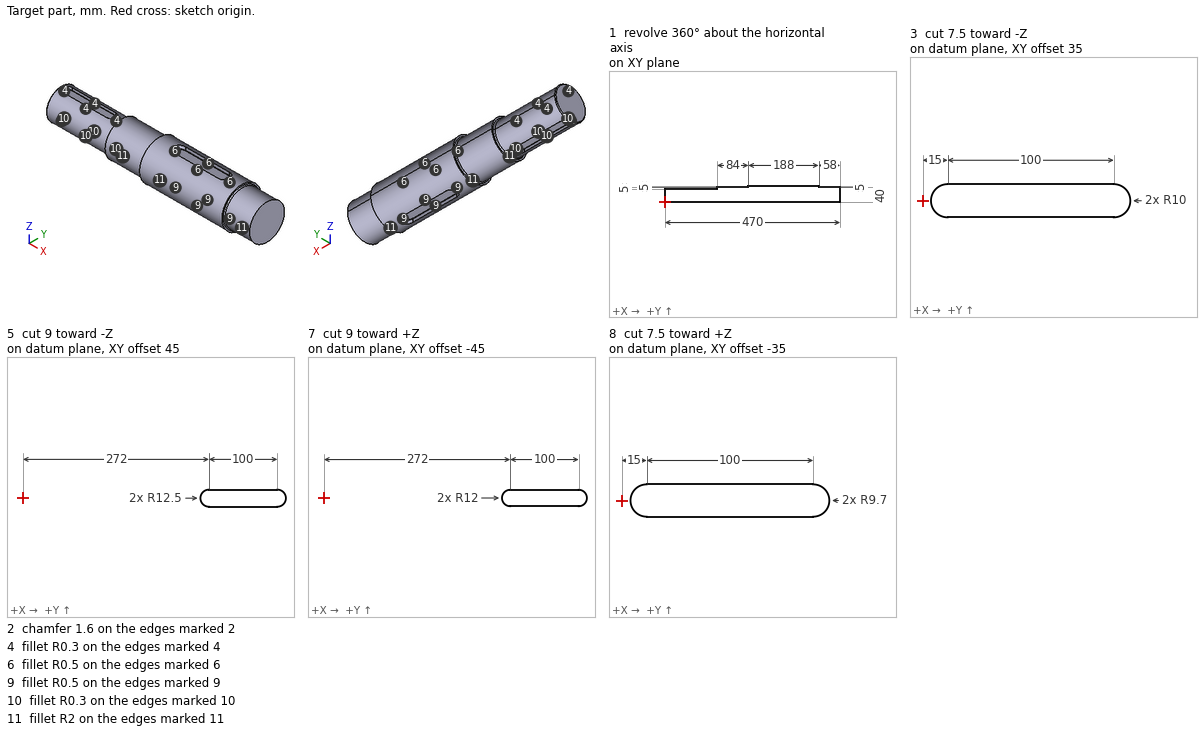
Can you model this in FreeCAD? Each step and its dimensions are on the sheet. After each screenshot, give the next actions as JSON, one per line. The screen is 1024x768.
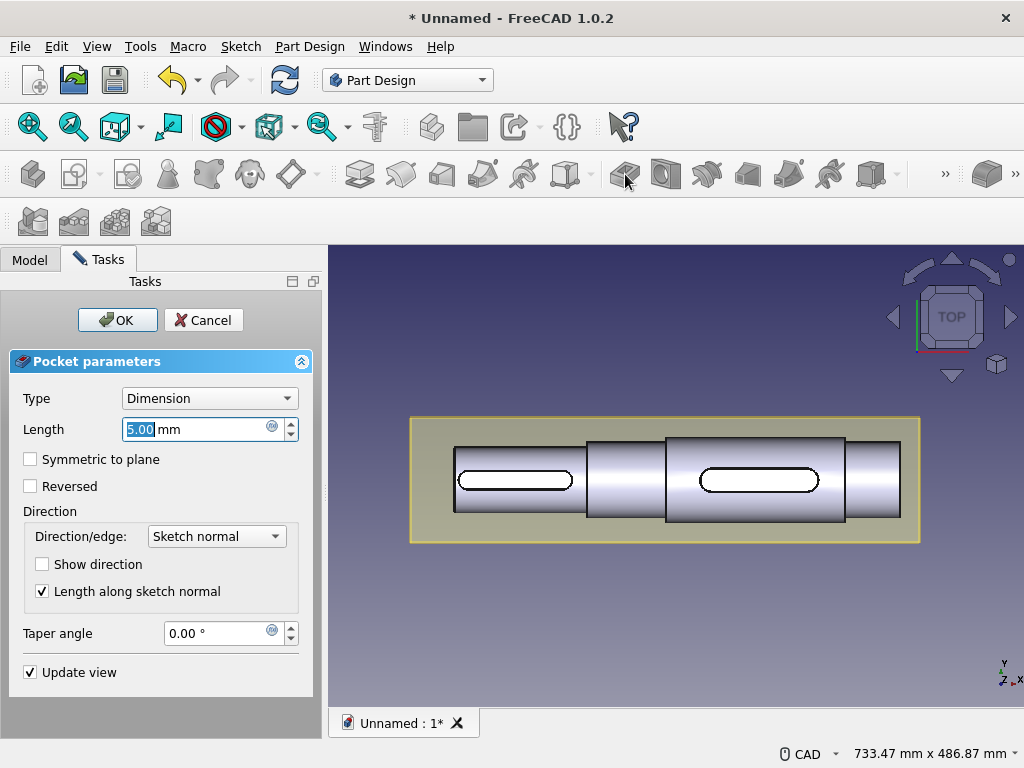
{"action": "type", "text": "9"}
{"action": "key", "text": "Tab"}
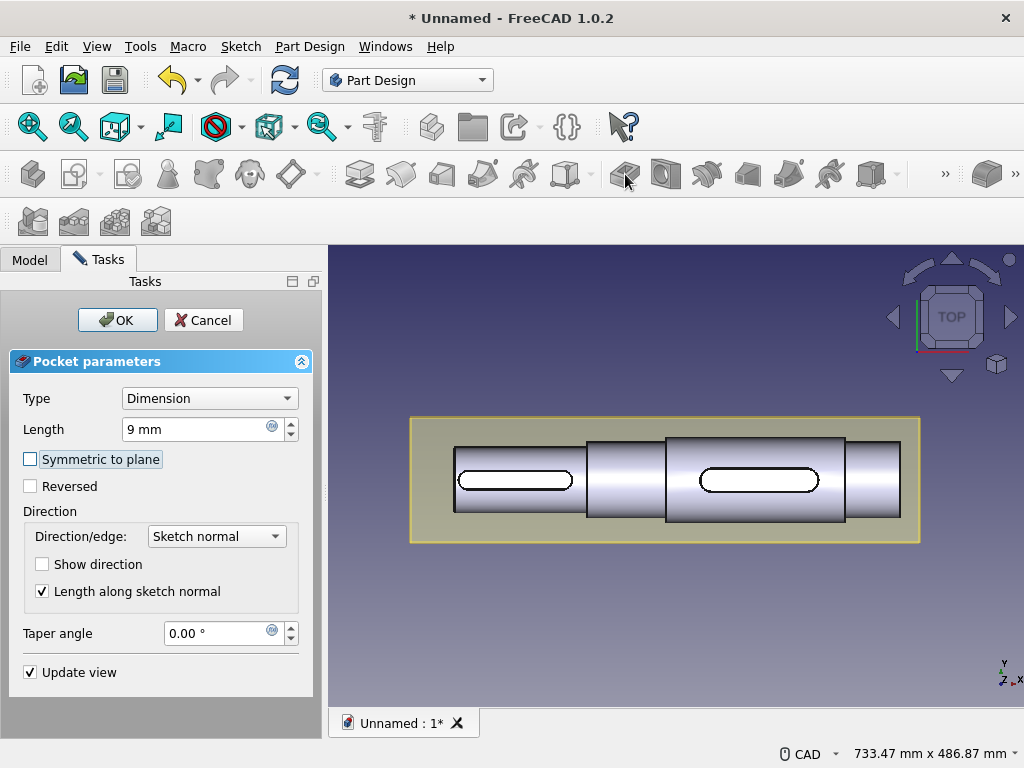
{"action": "left_click", "coordinate": [31, 486]}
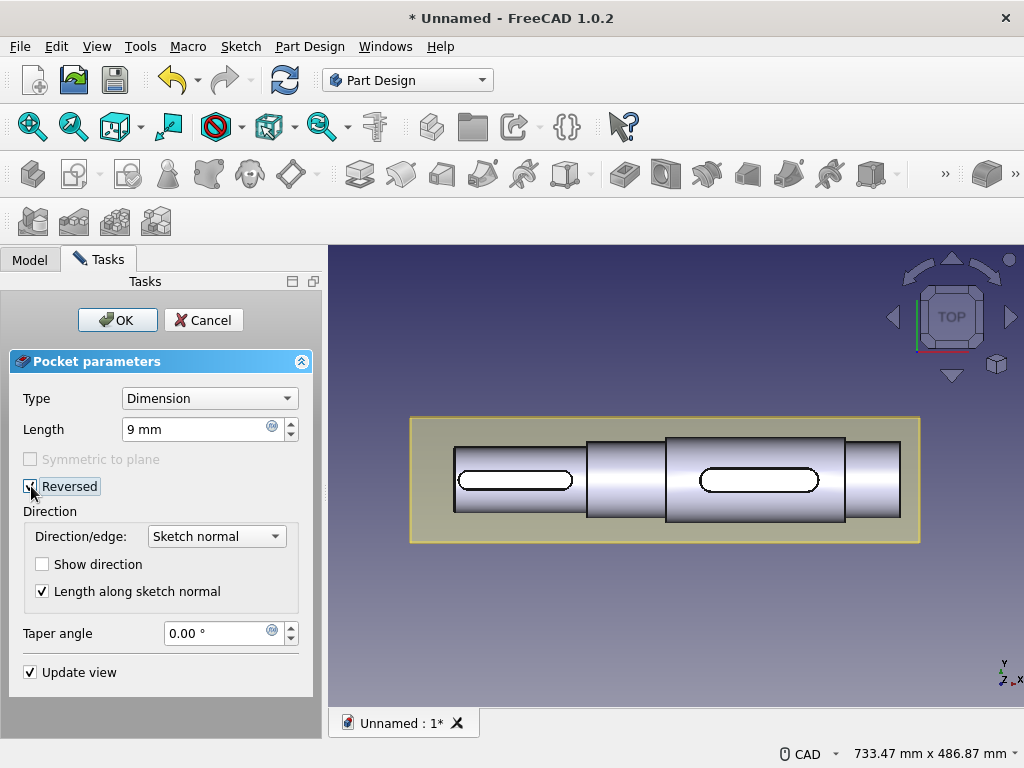
{"action": "left_click", "coordinate": [118, 320]}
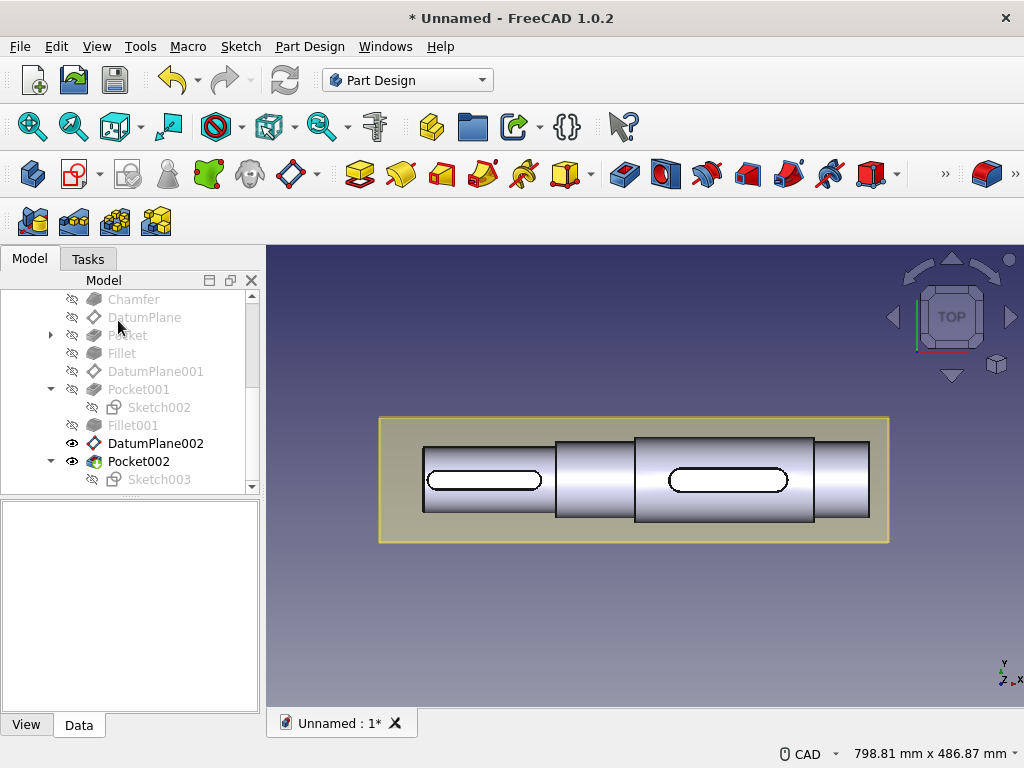
{"action": "left_click", "coordinate": [117, 443]}
{"action": "key", "text": "space"}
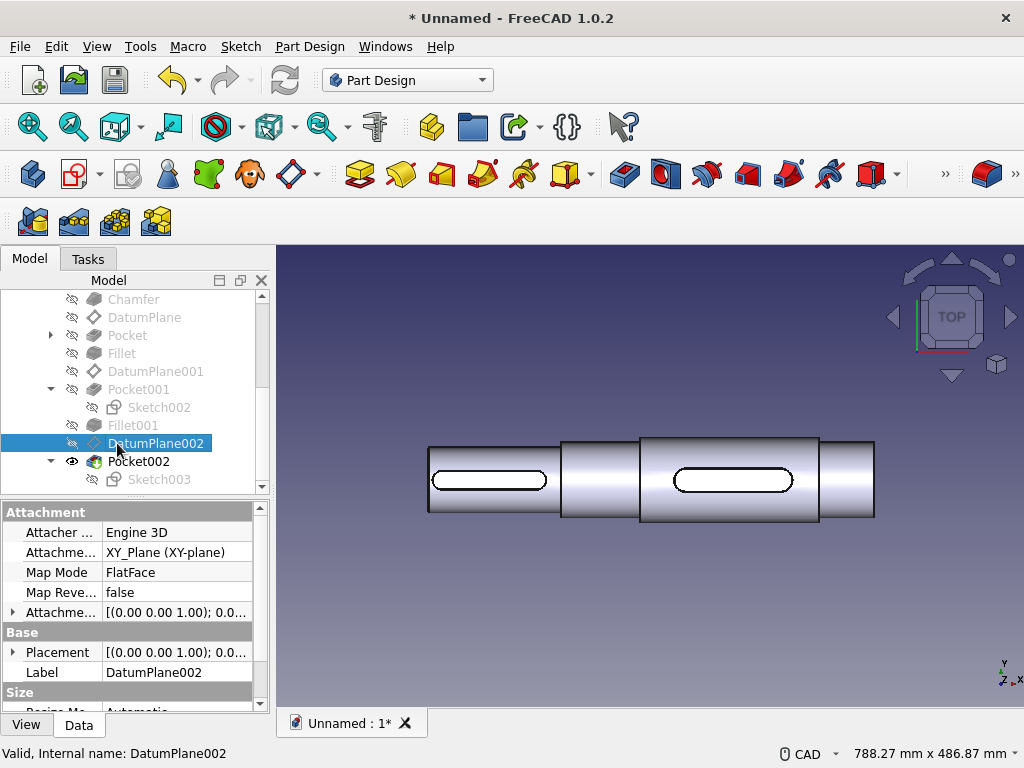
{"action": "scroll", "coordinate": [141, 385], "scroll_direction": "down", "scroll_amount": 3}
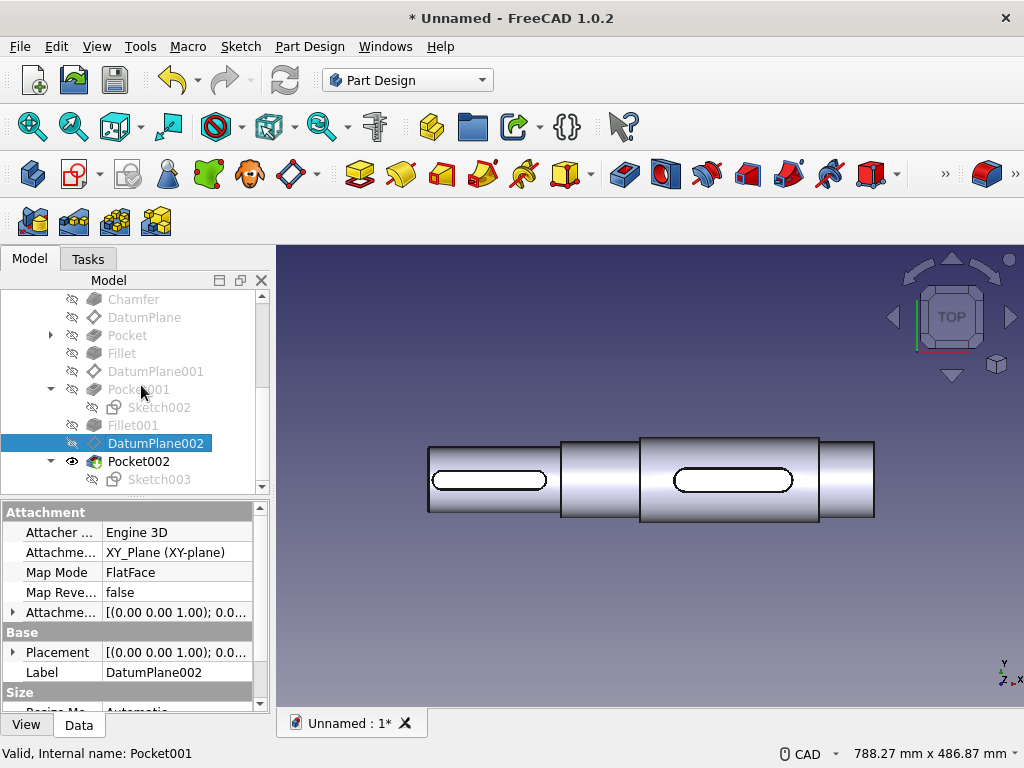
{"action": "scroll", "coordinate": [141, 385], "scroll_direction": "up", "scroll_amount": 15}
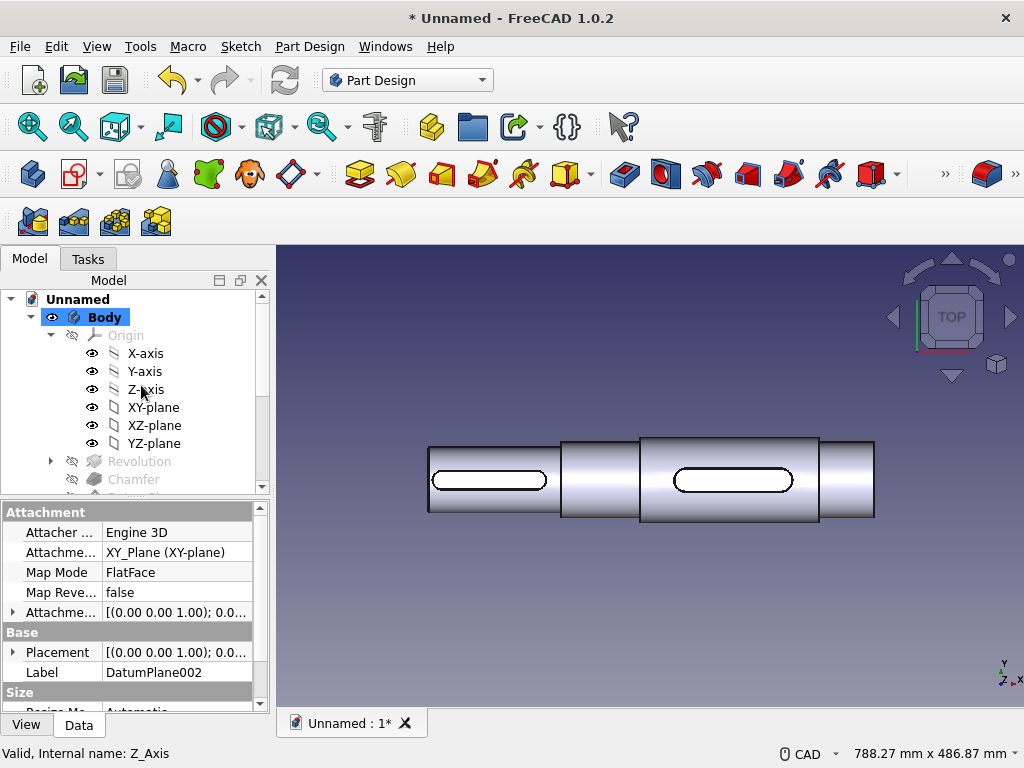
{"action": "left_click", "coordinate": [137, 407]}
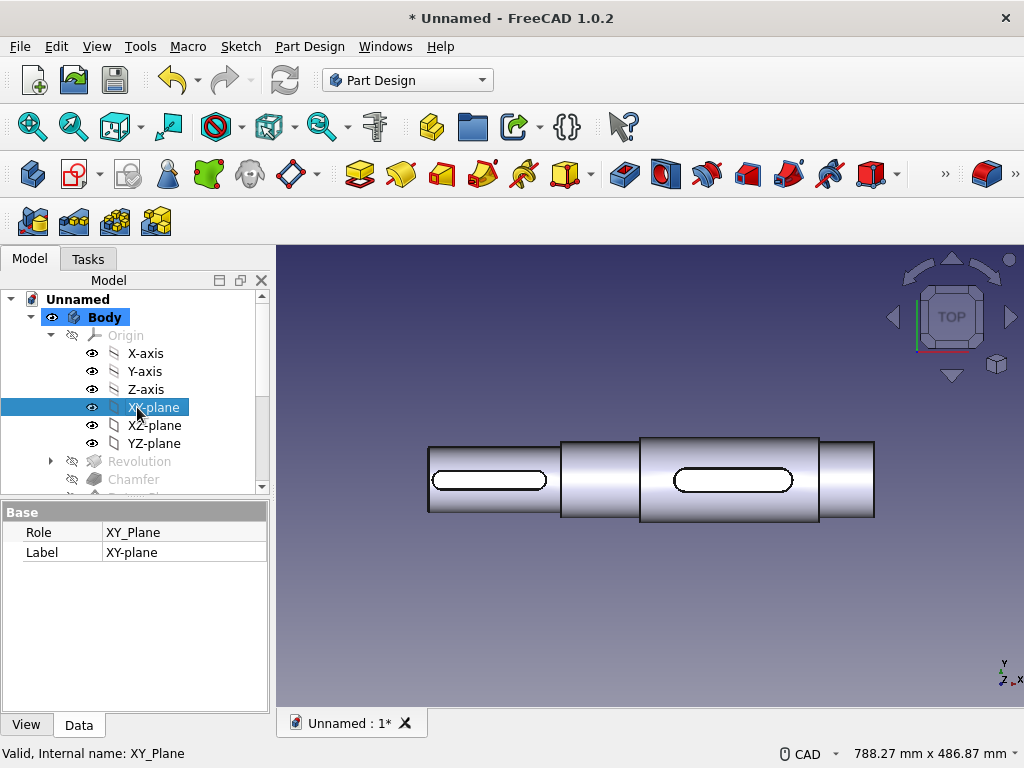
{"action": "left_click", "coordinate": [290, 174]}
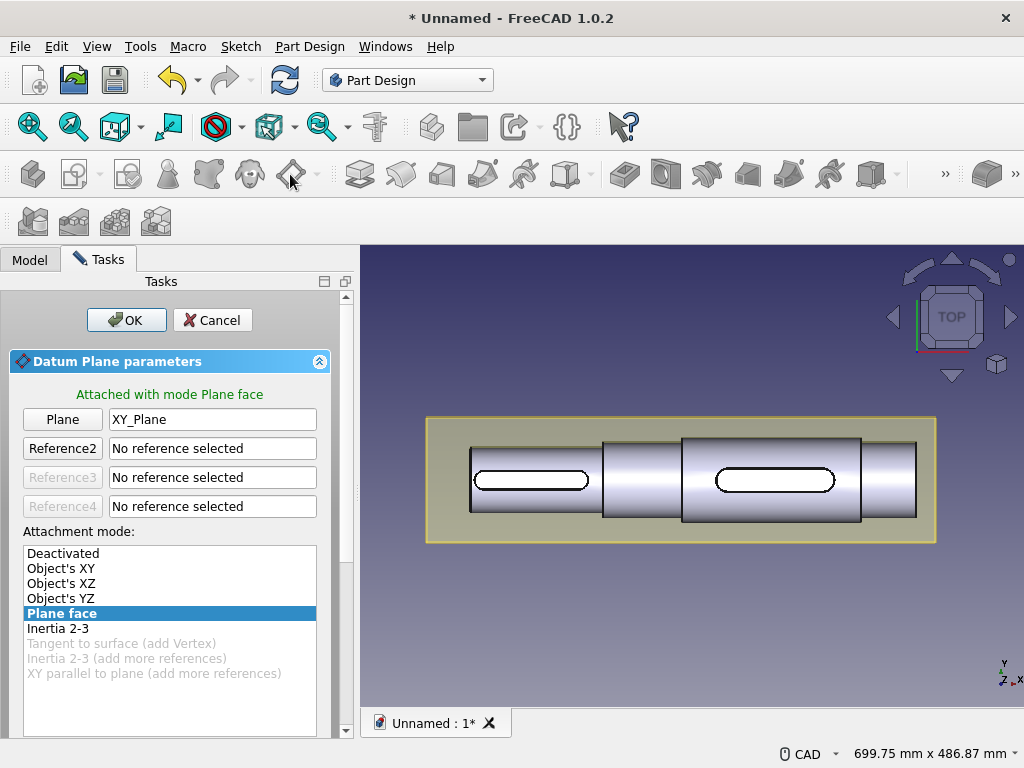
{"action": "scroll", "coordinate": [346, 514], "scroll_direction": "down", "scroll_amount": 4}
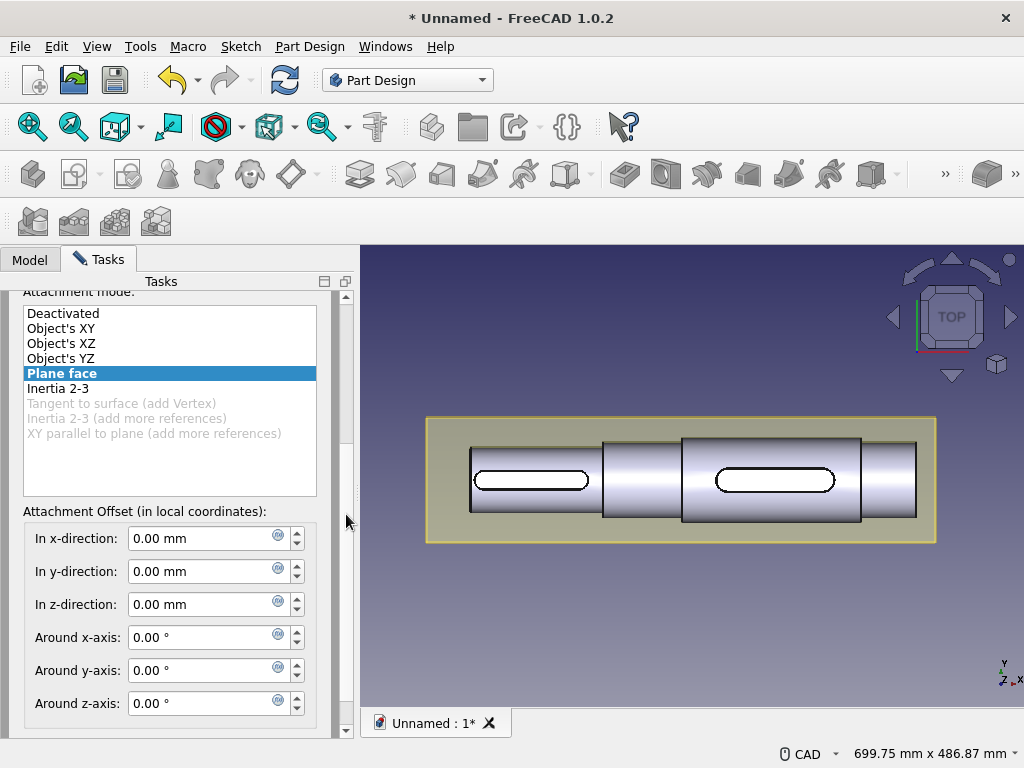
{"action": "triple_click", "coordinate": [210, 604]}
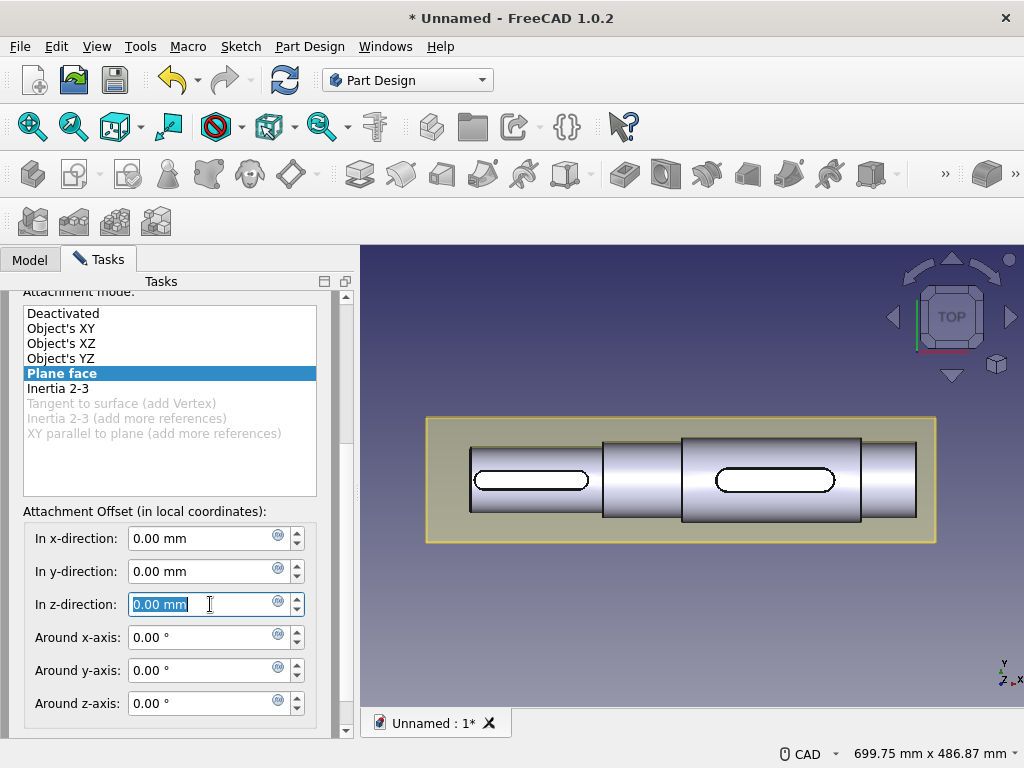
{"action": "type", "text": "-35"}
{"action": "key", "text": "Tab"}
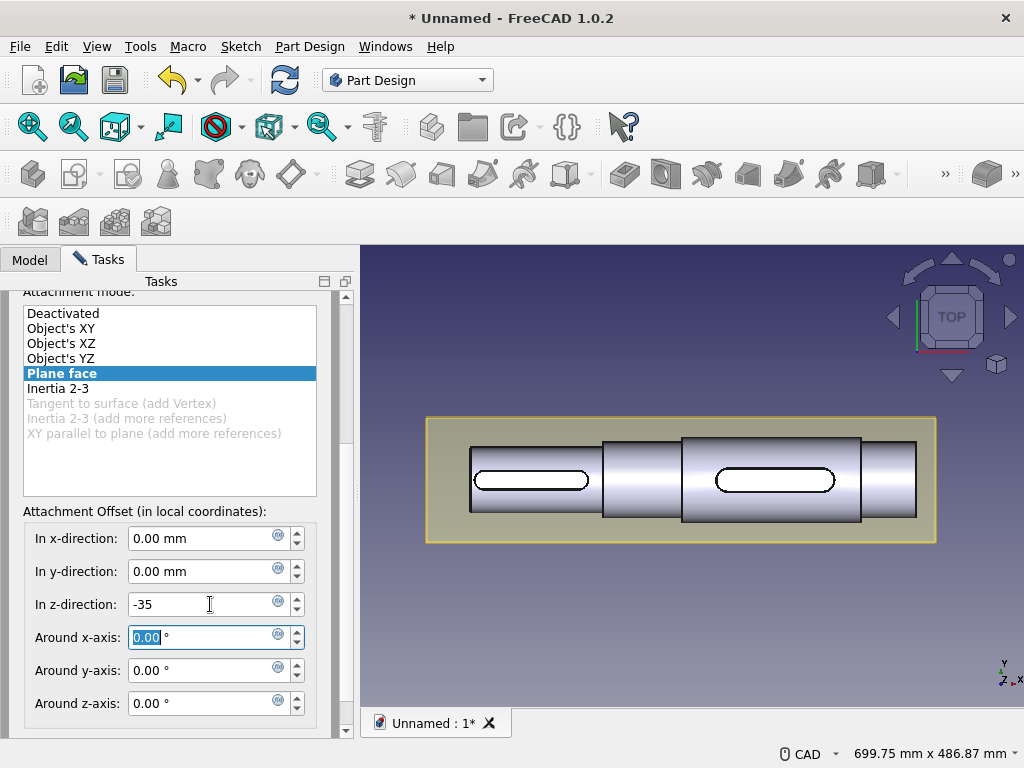
{"action": "scroll", "coordinate": [346, 514], "scroll_direction": "up", "scroll_amount": 5}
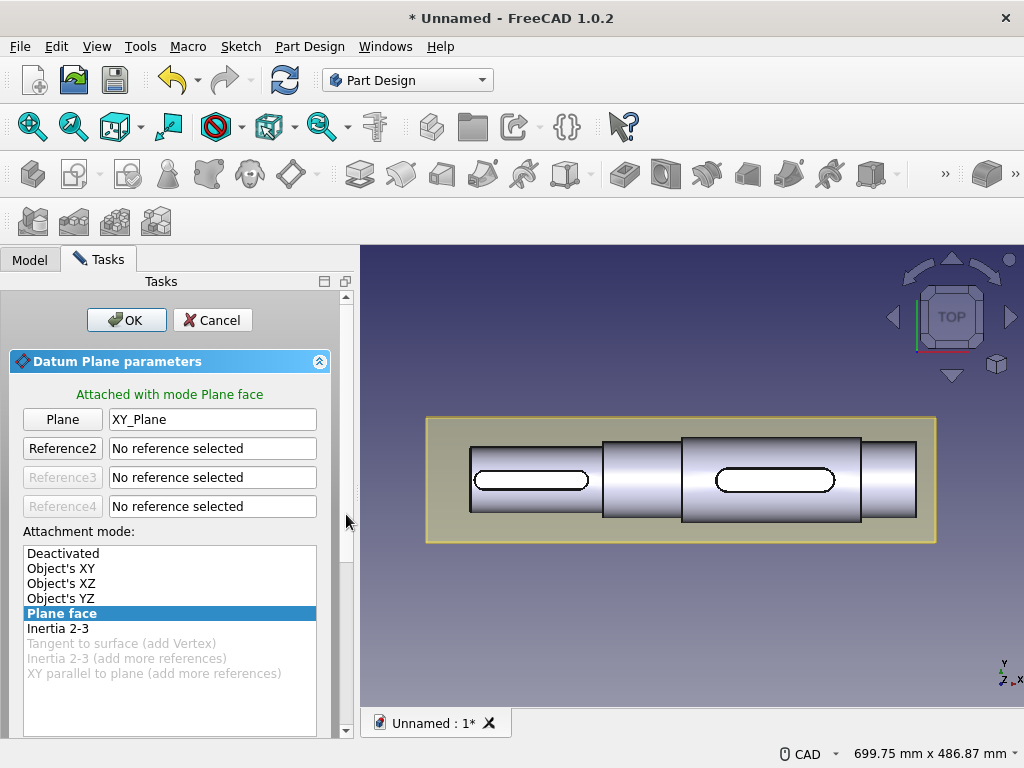
{"action": "left_click", "coordinate": [127, 320]}